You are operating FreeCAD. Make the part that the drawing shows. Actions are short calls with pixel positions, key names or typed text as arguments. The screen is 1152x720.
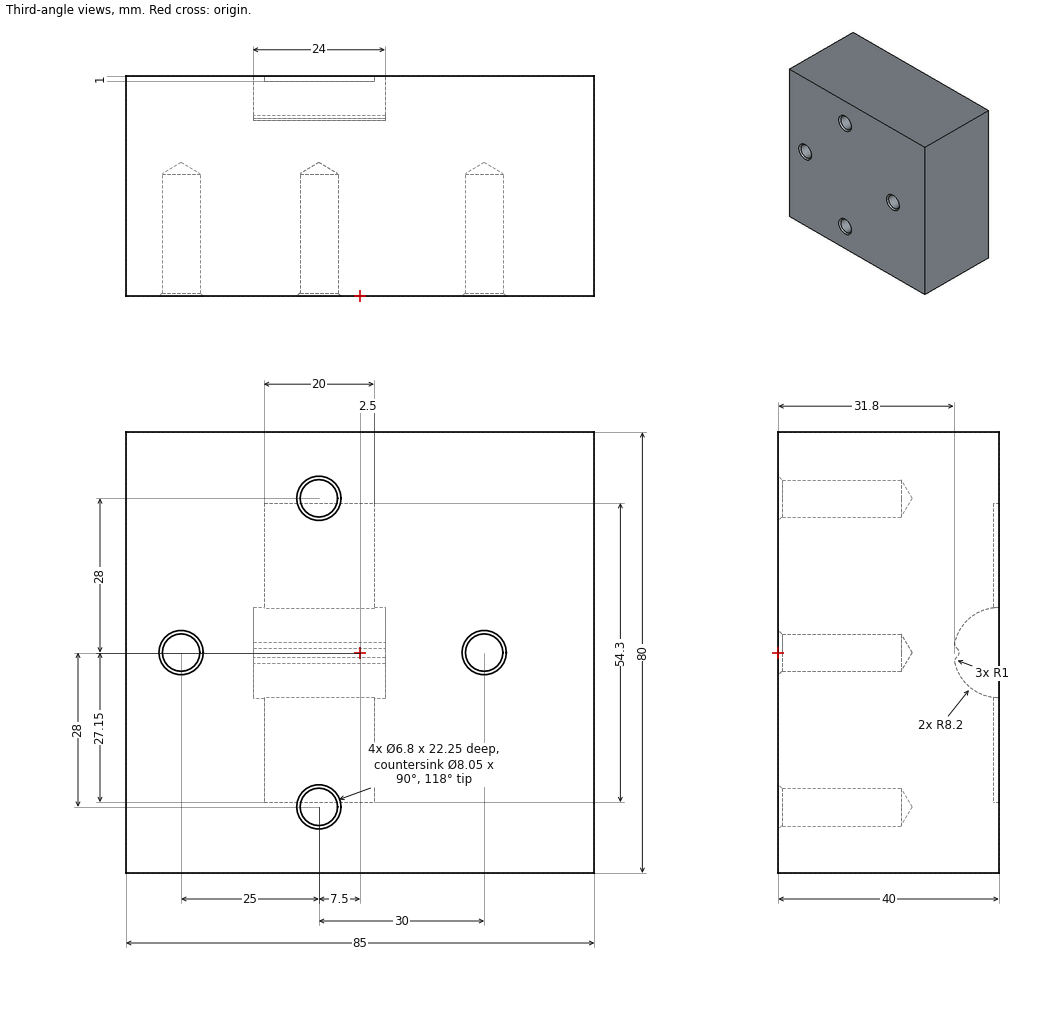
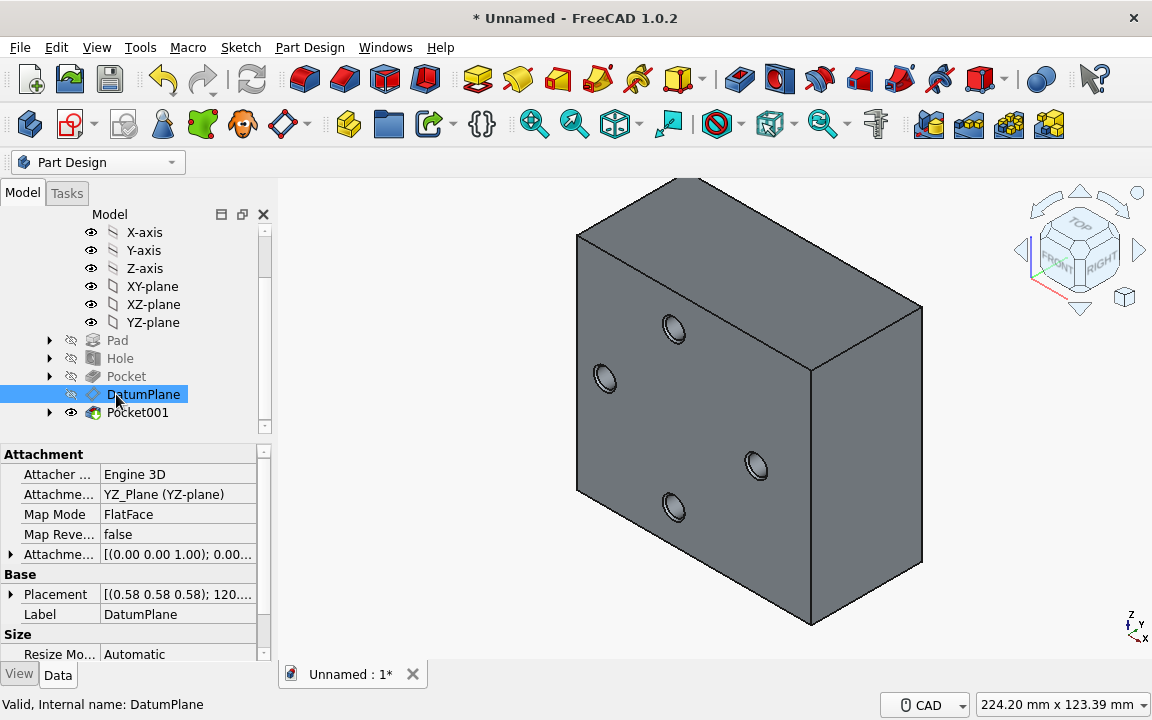
click(536, 124)